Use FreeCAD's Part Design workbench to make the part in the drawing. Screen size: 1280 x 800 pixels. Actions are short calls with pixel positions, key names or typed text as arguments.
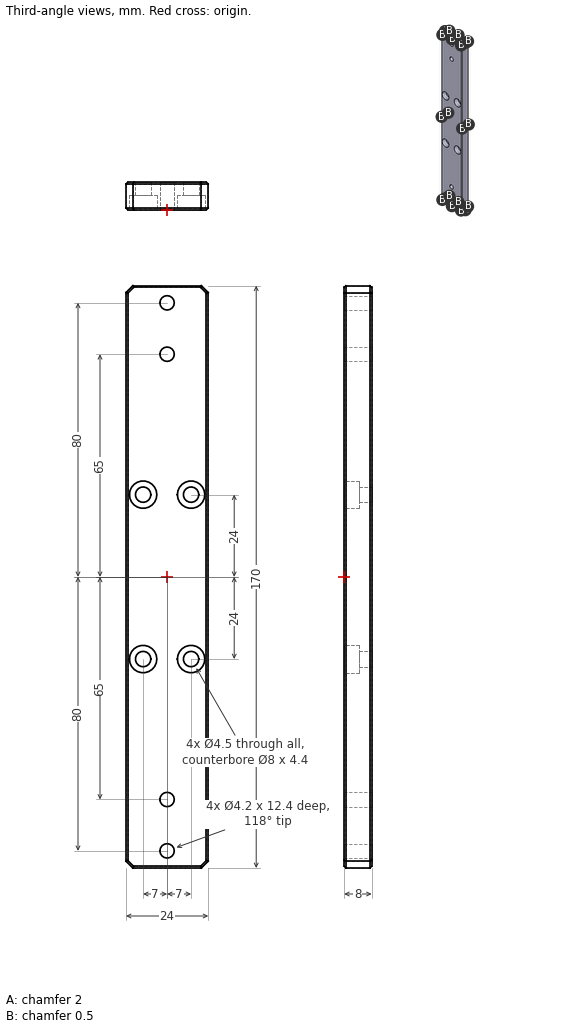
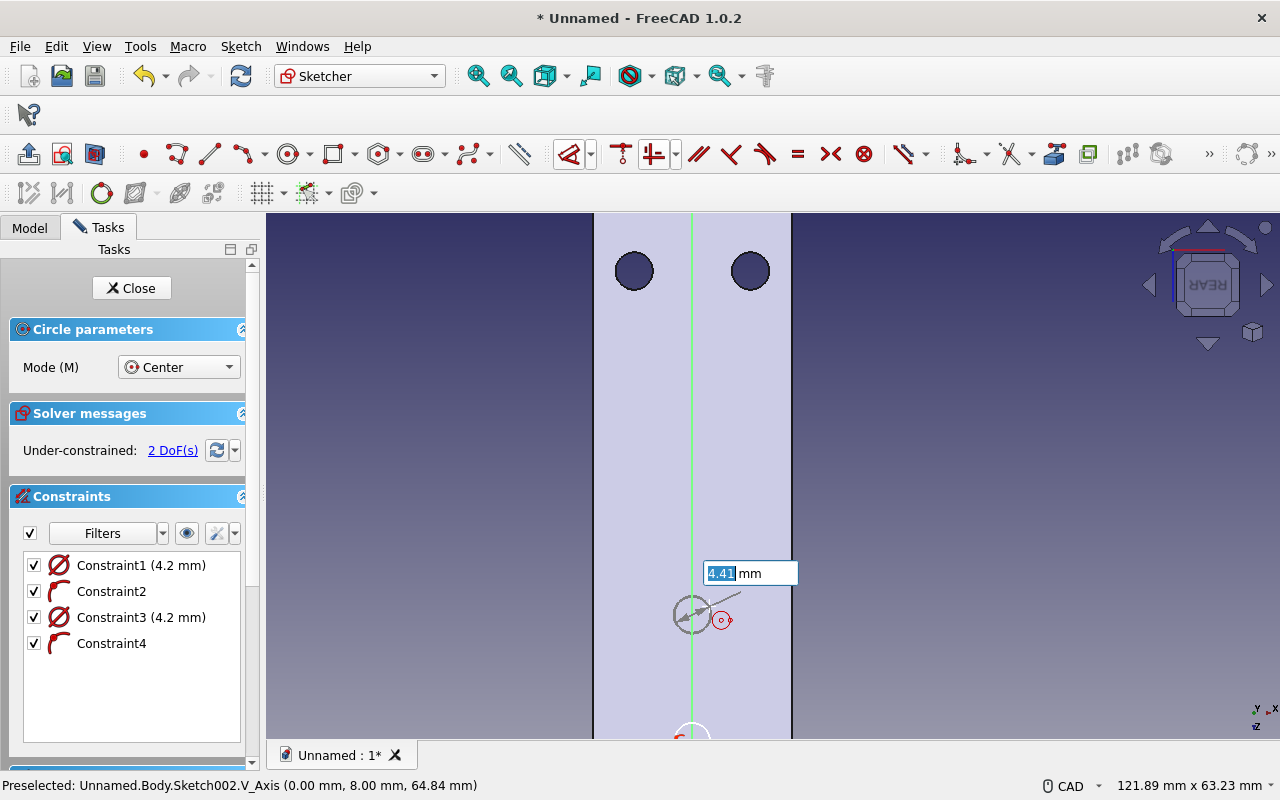
text(4.2)
key(Return)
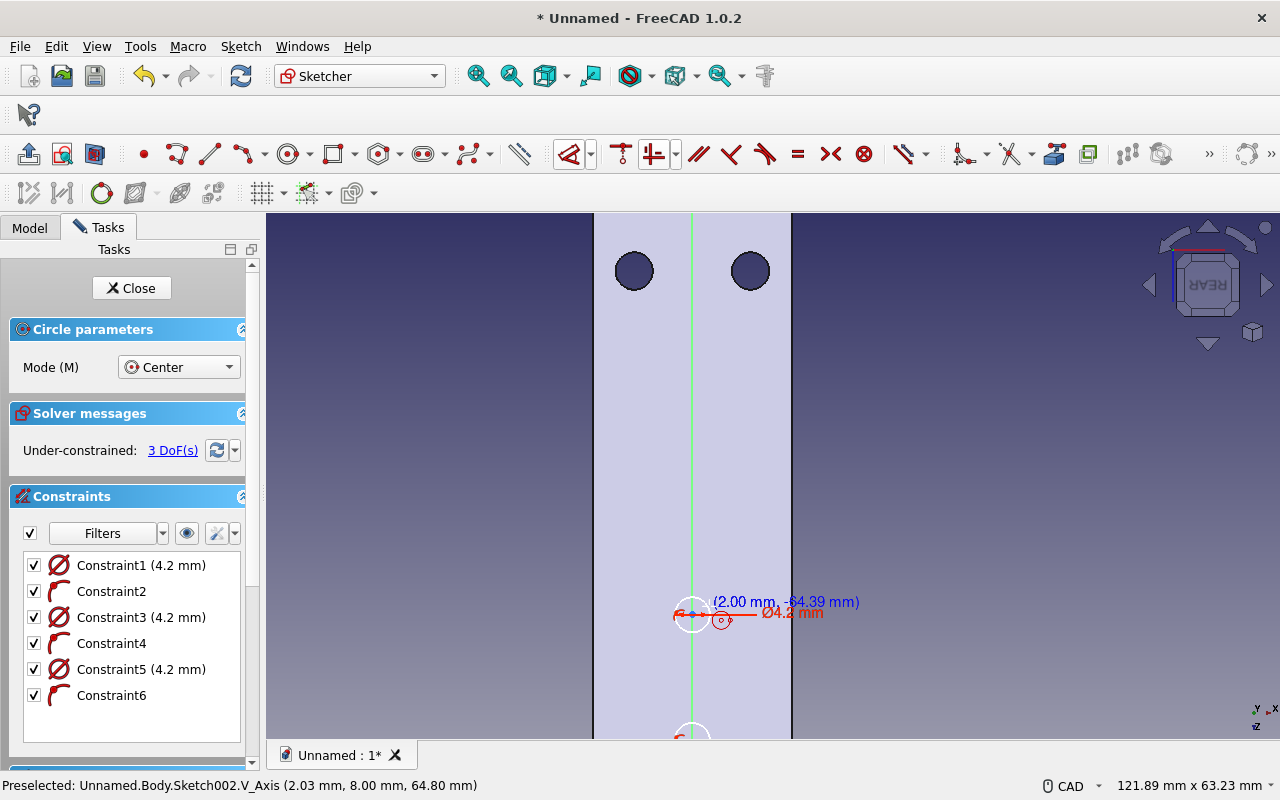
scroll(708, 608, down, 7)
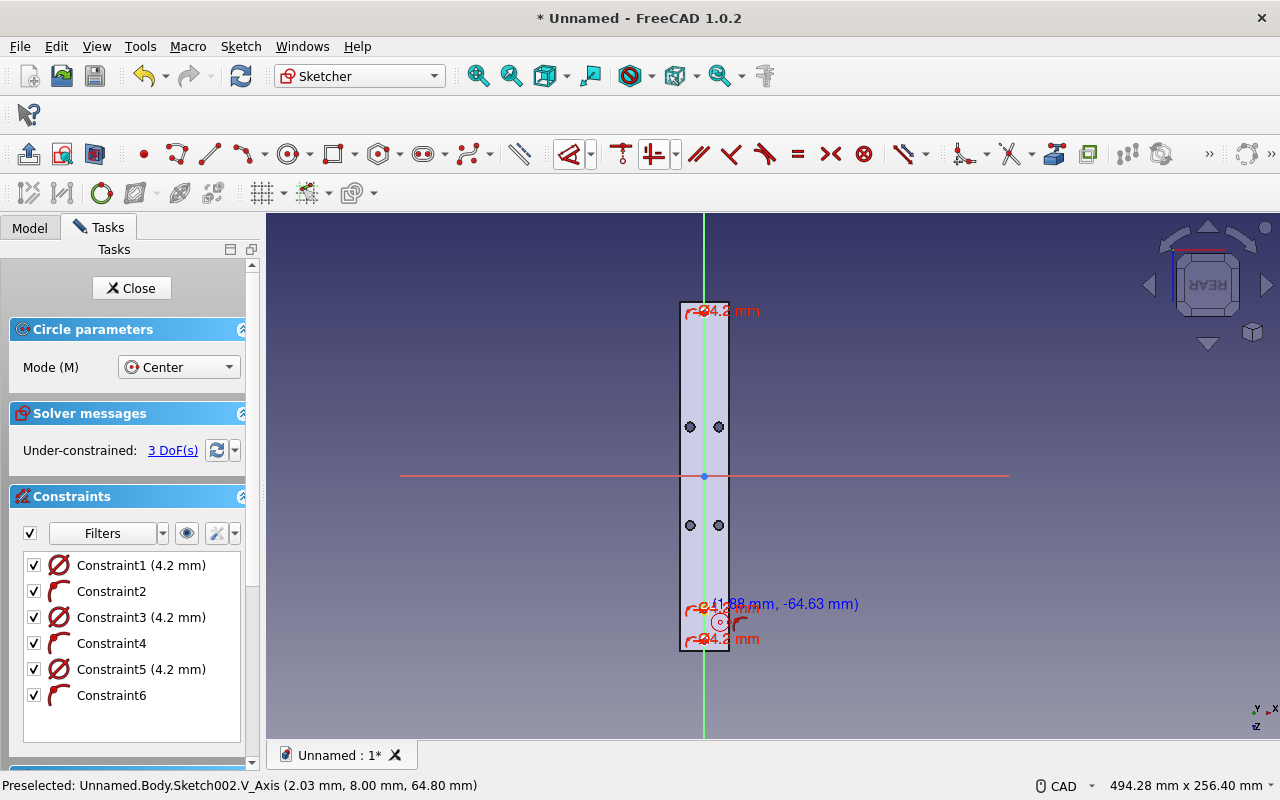
scroll(704, 343, up, 9)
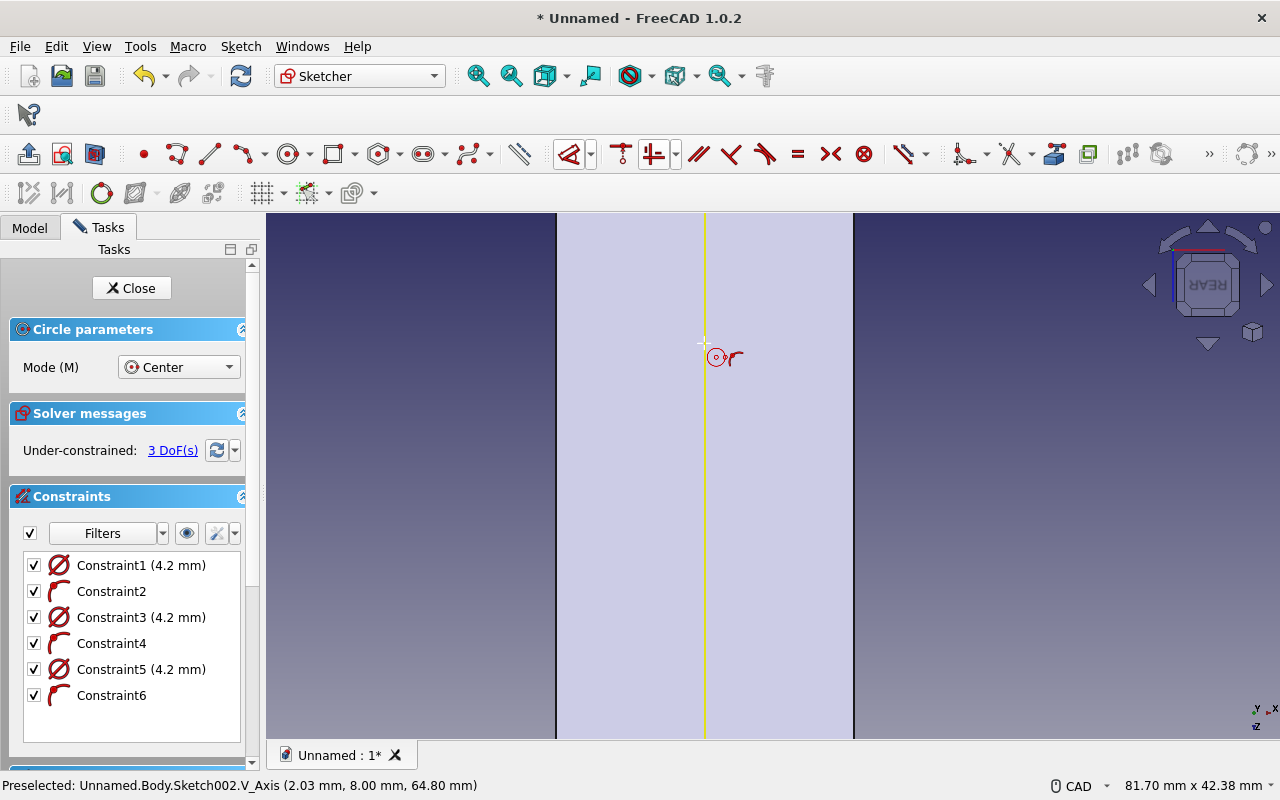
scroll(704, 343, down, 9)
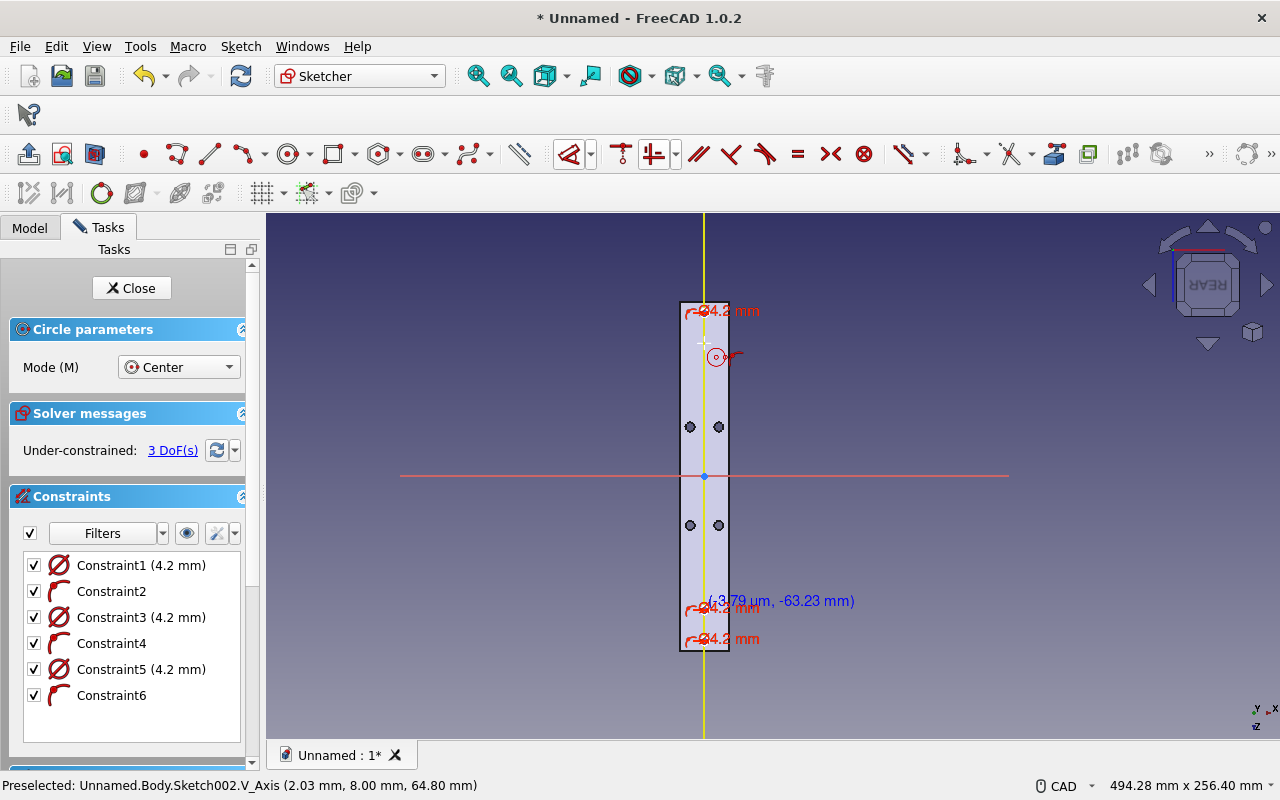
click(704, 343)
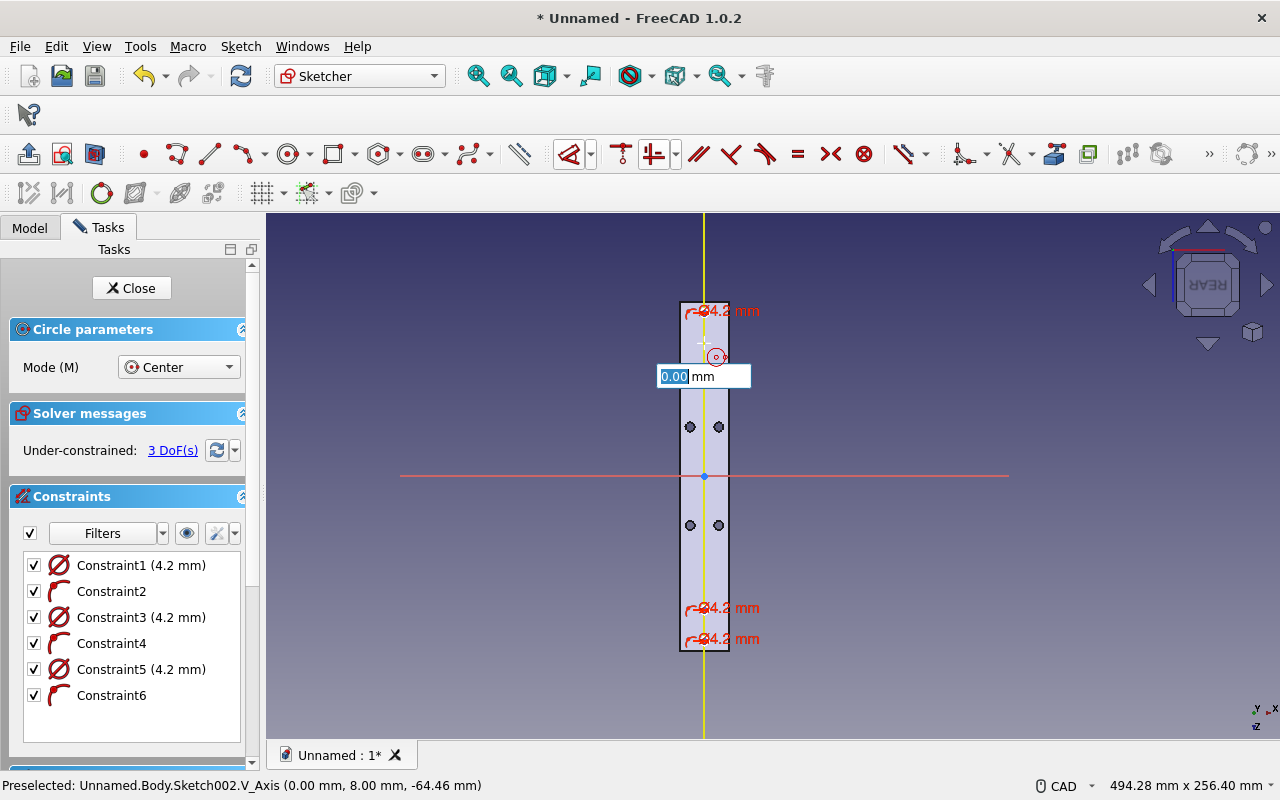
scroll(709, 341, up, 7)
move(706, 342)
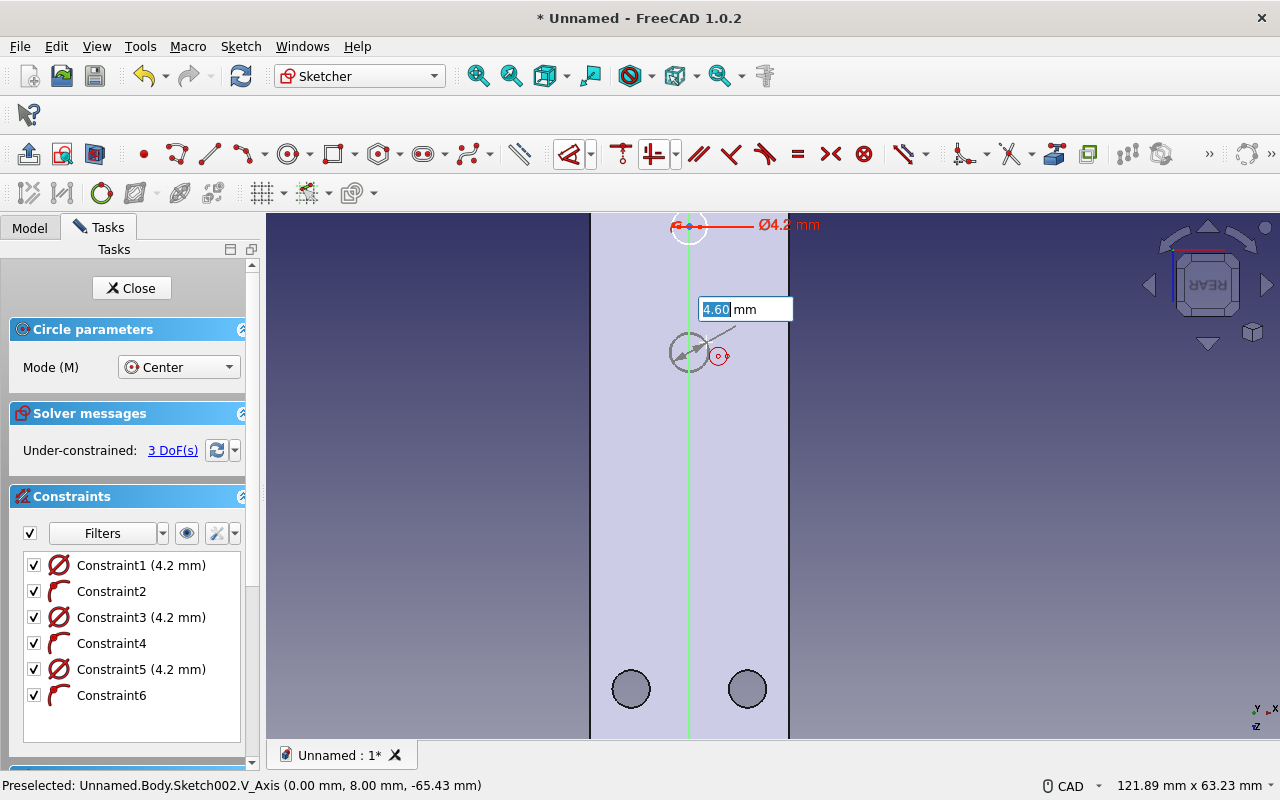
text(4.2)
key(Return)
key(Escape)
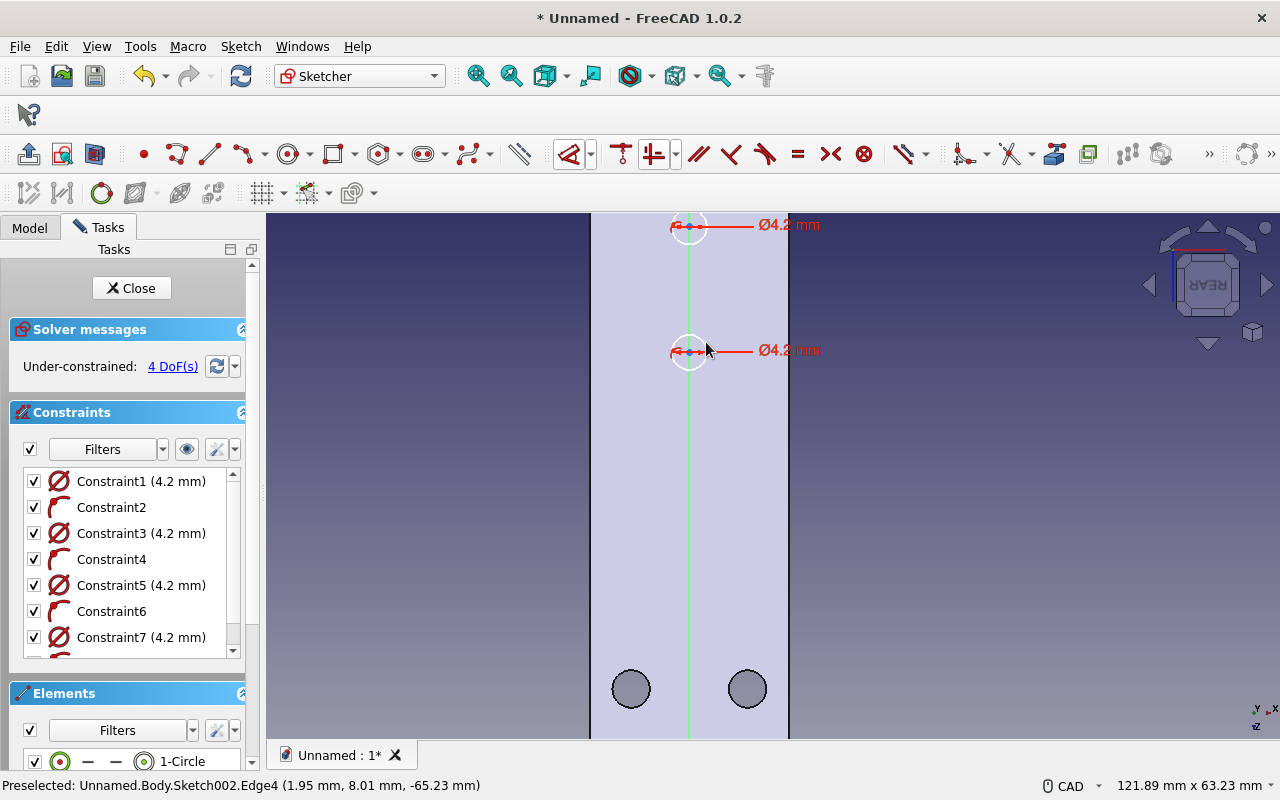
scroll(709, 341, down, 7)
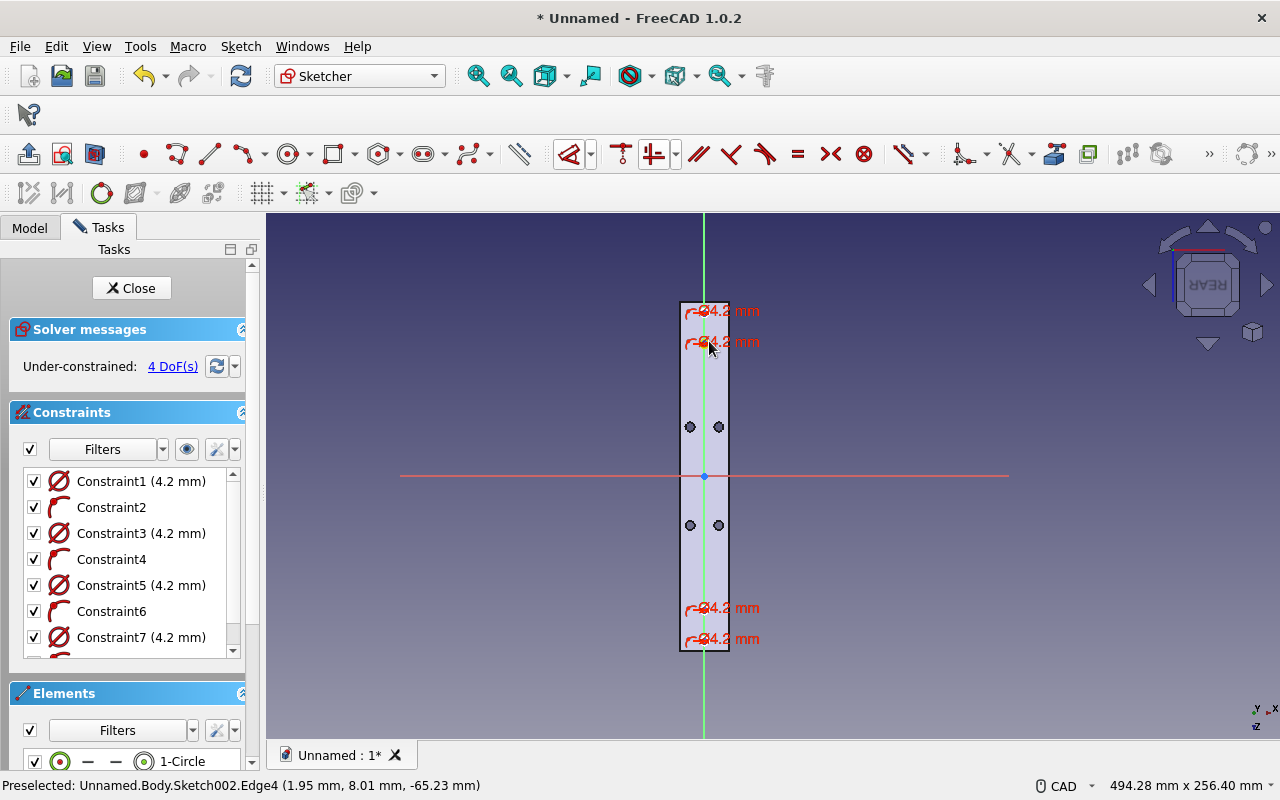
click(704, 313)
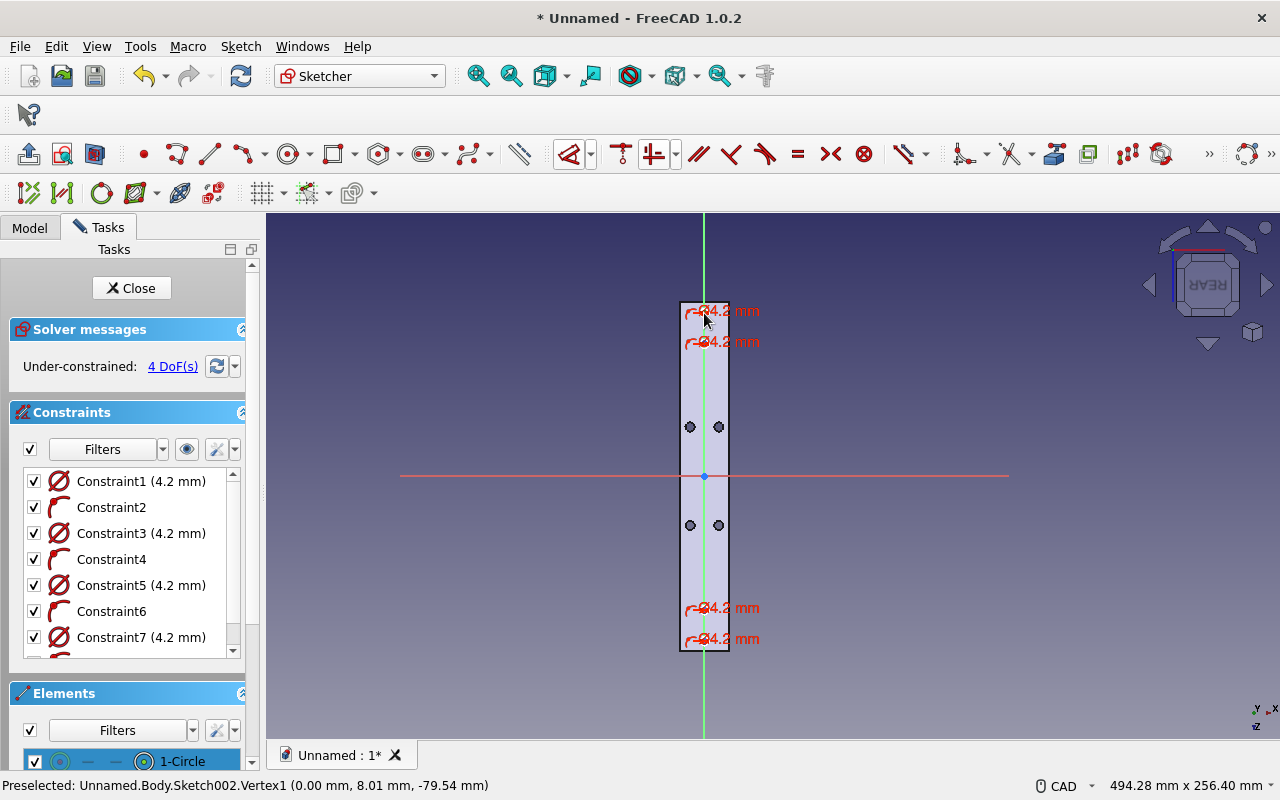
click(590, 154)